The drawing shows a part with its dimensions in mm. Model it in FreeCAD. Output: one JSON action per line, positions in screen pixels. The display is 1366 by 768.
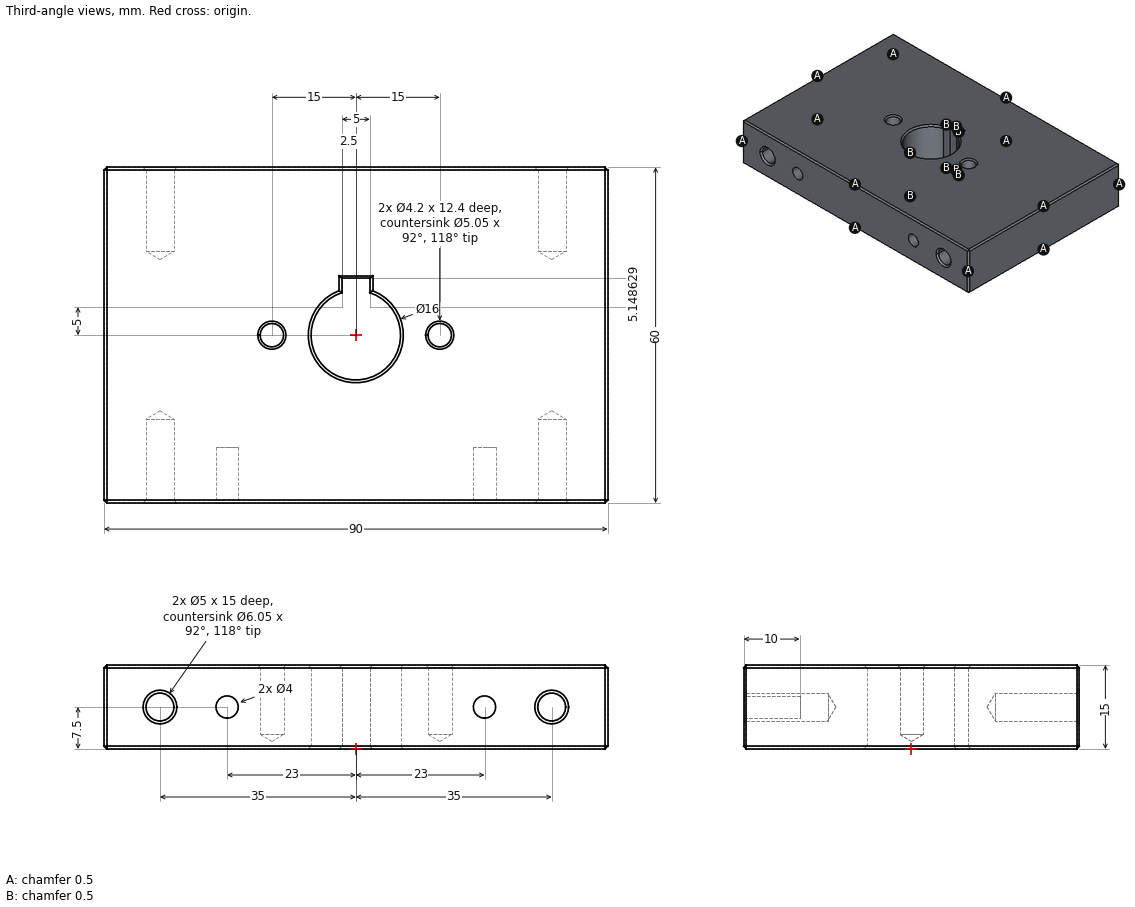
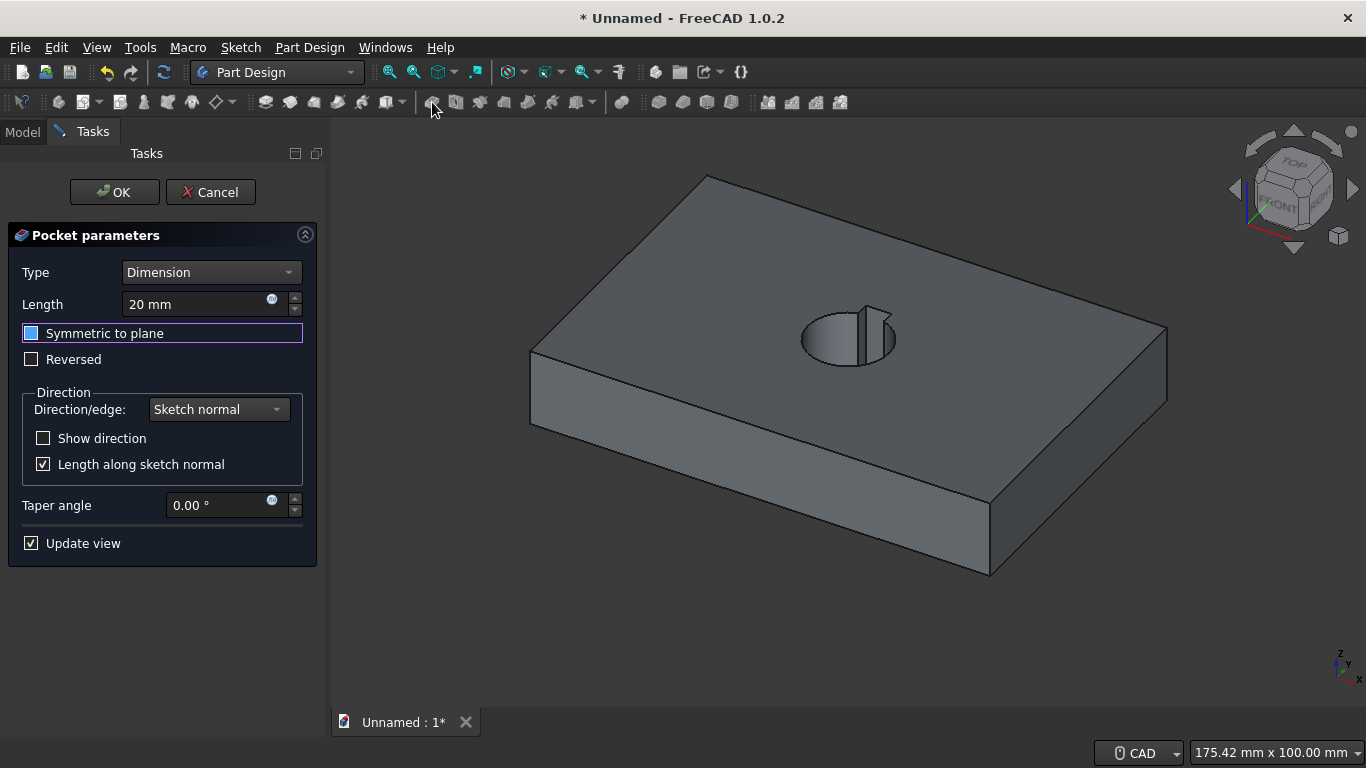
{"action": "left_click", "coordinate": [115, 192]}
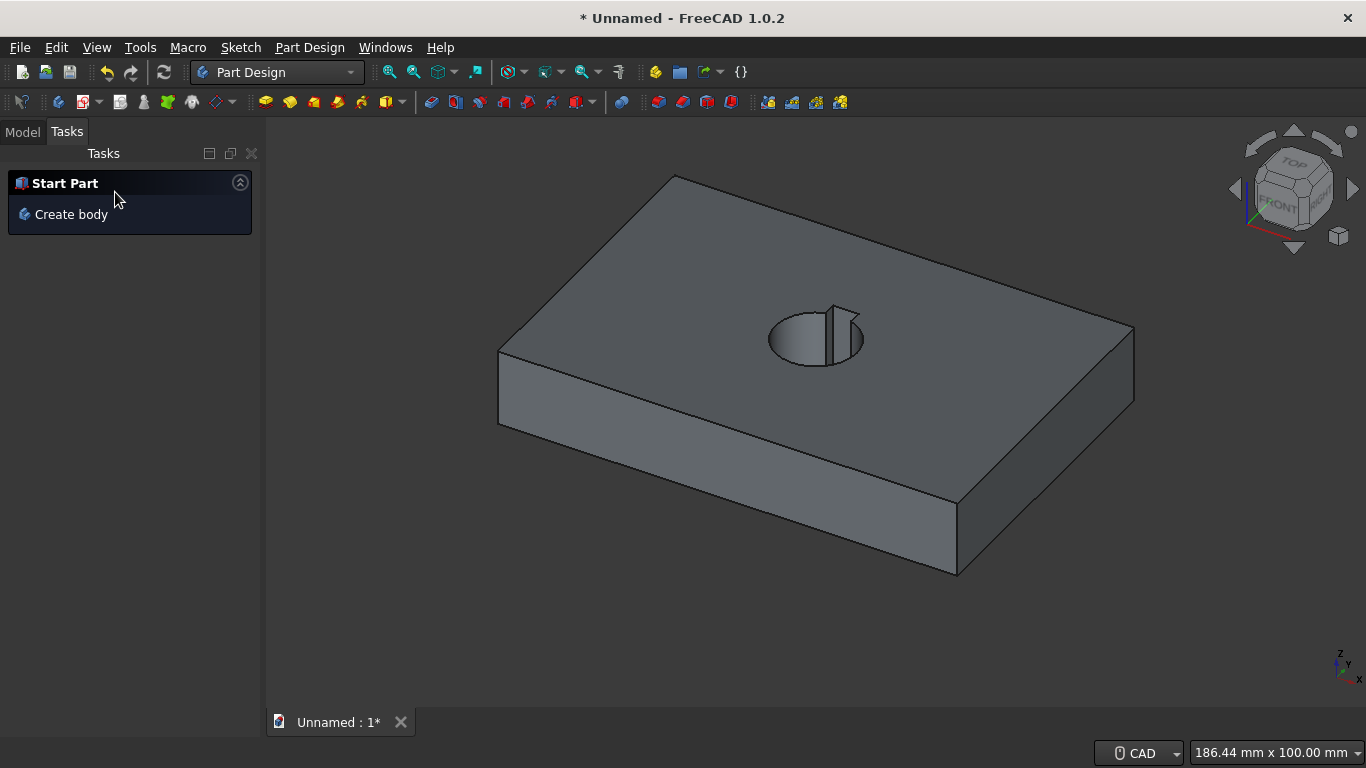
{"action": "left_click", "coordinate": [659, 320]}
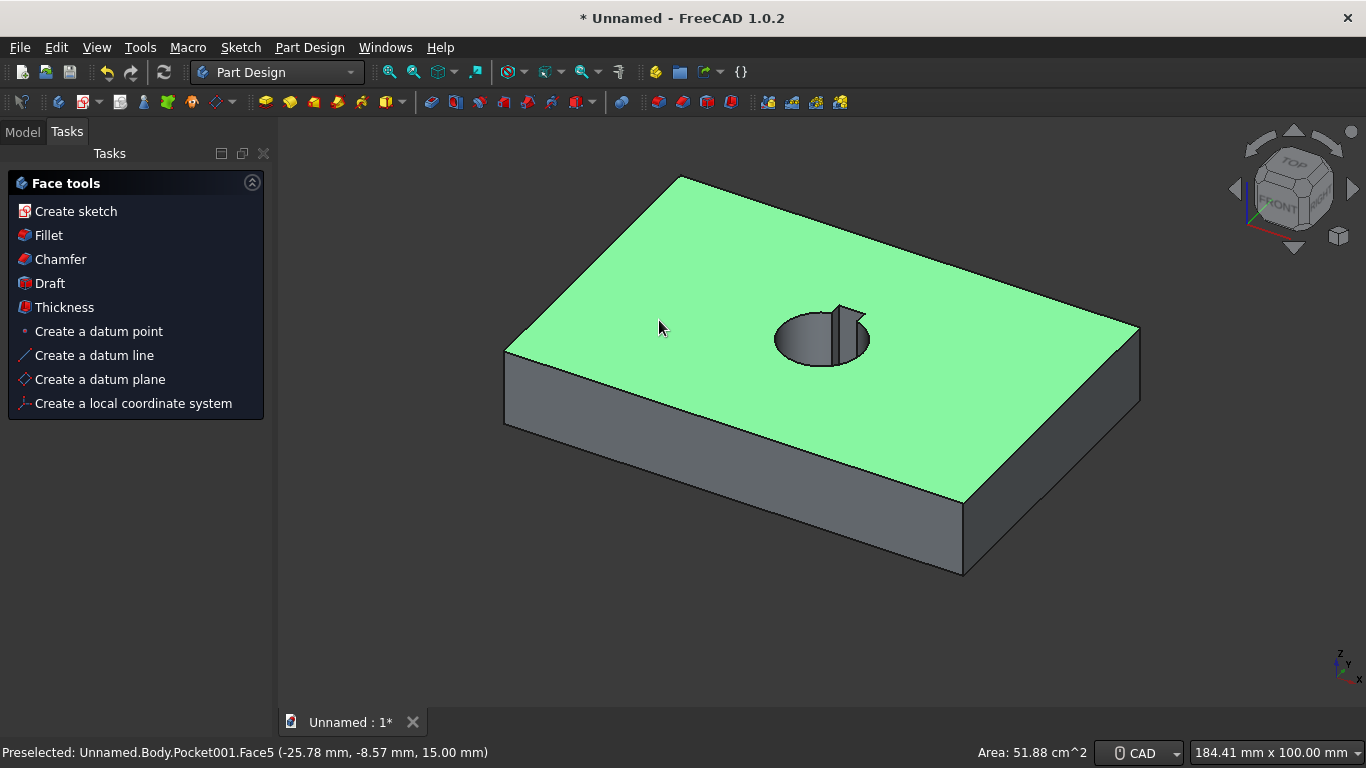
{"action": "left_click", "coordinate": [84, 102]}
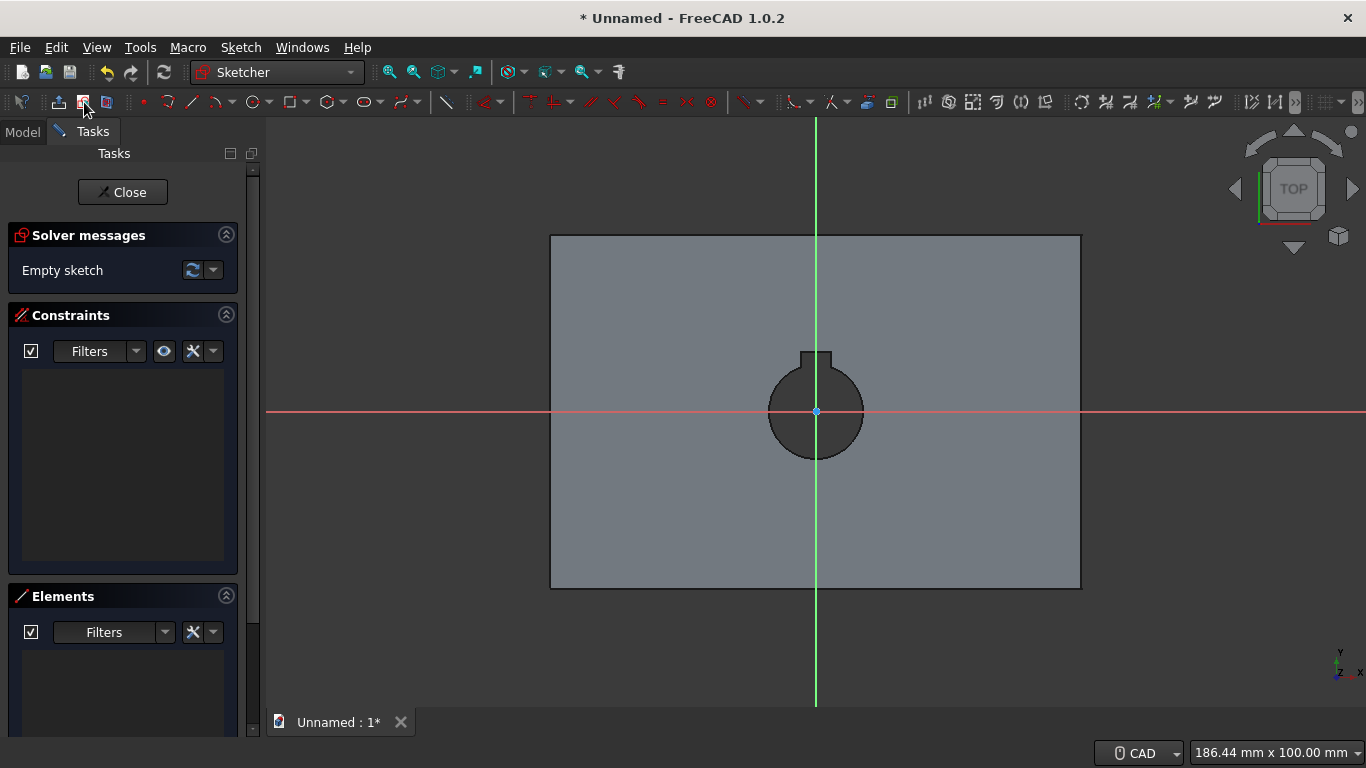
{"action": "scroll", "coordinate": [846, 412], "scroll_direction": "up", "scroll_amount": 6}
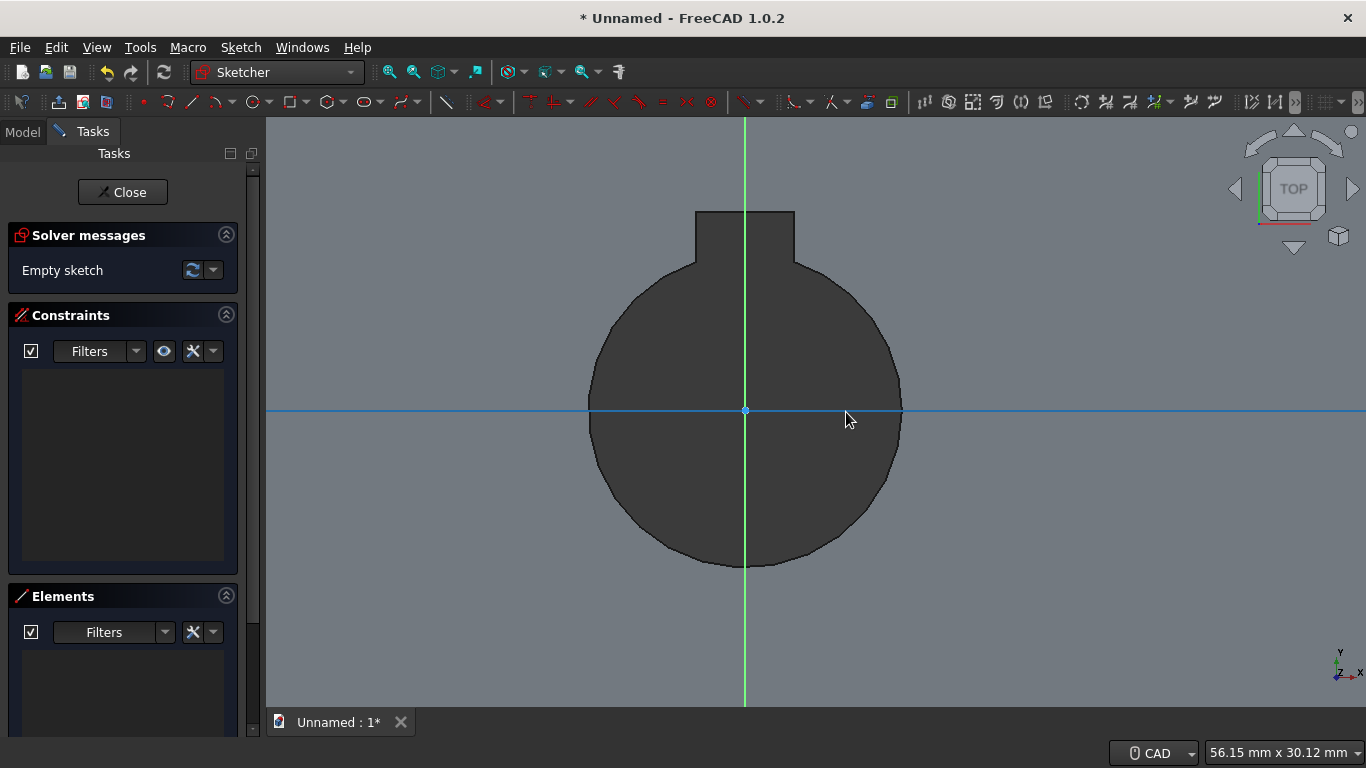
{"action": "left_click", "coordinate": [254, 102]}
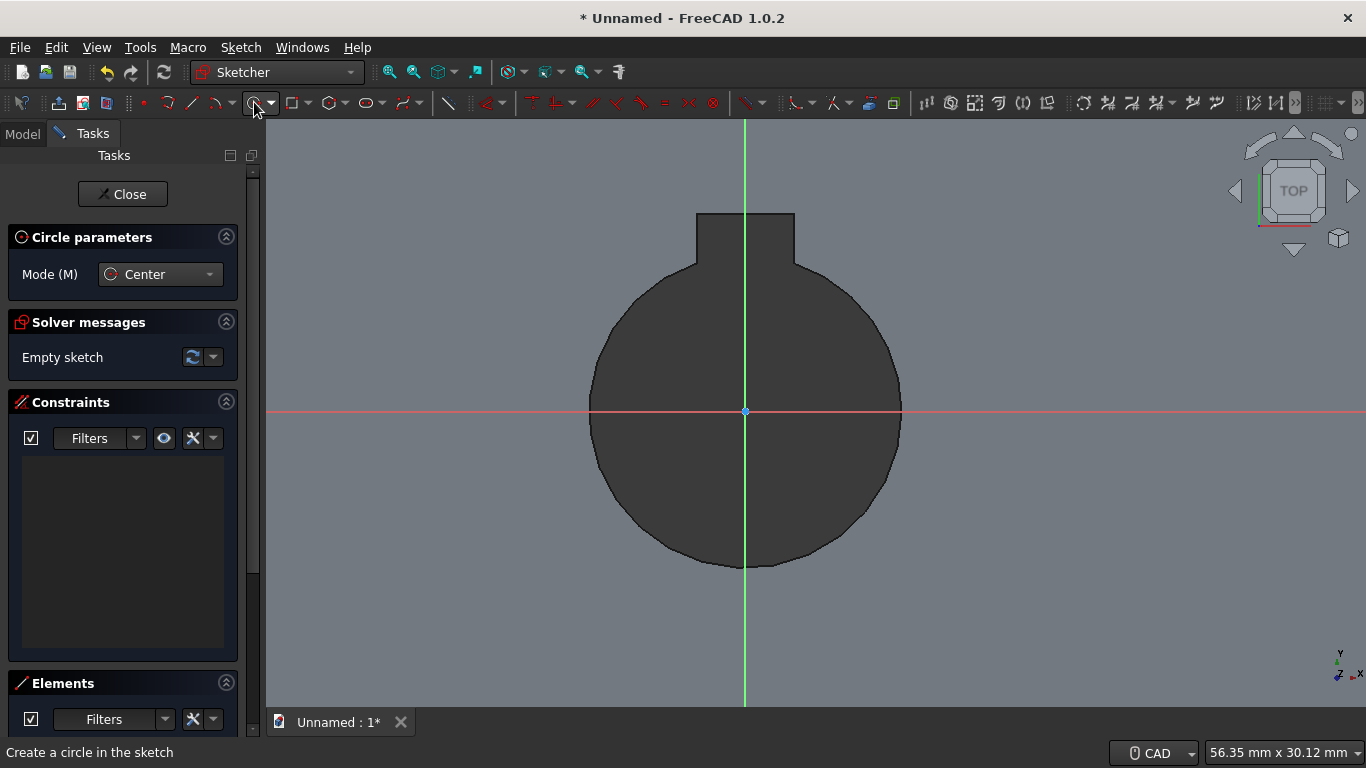
{"action": "left_click", "coordinate": [1038, 412]}
{"action": "mouse_move", "coordinate": [1067, 383]}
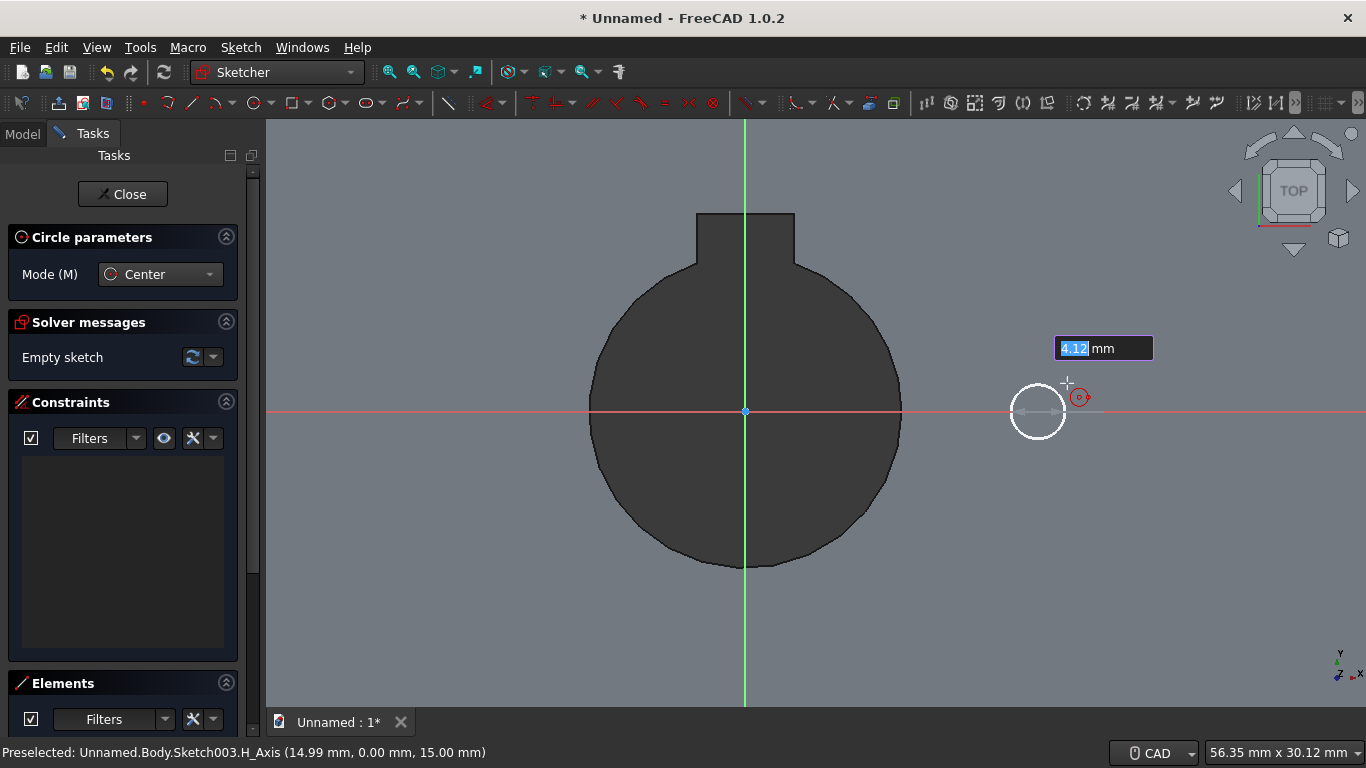
{"action": "type", "text": "4.2"}
{"action": "key", "text": "Return"}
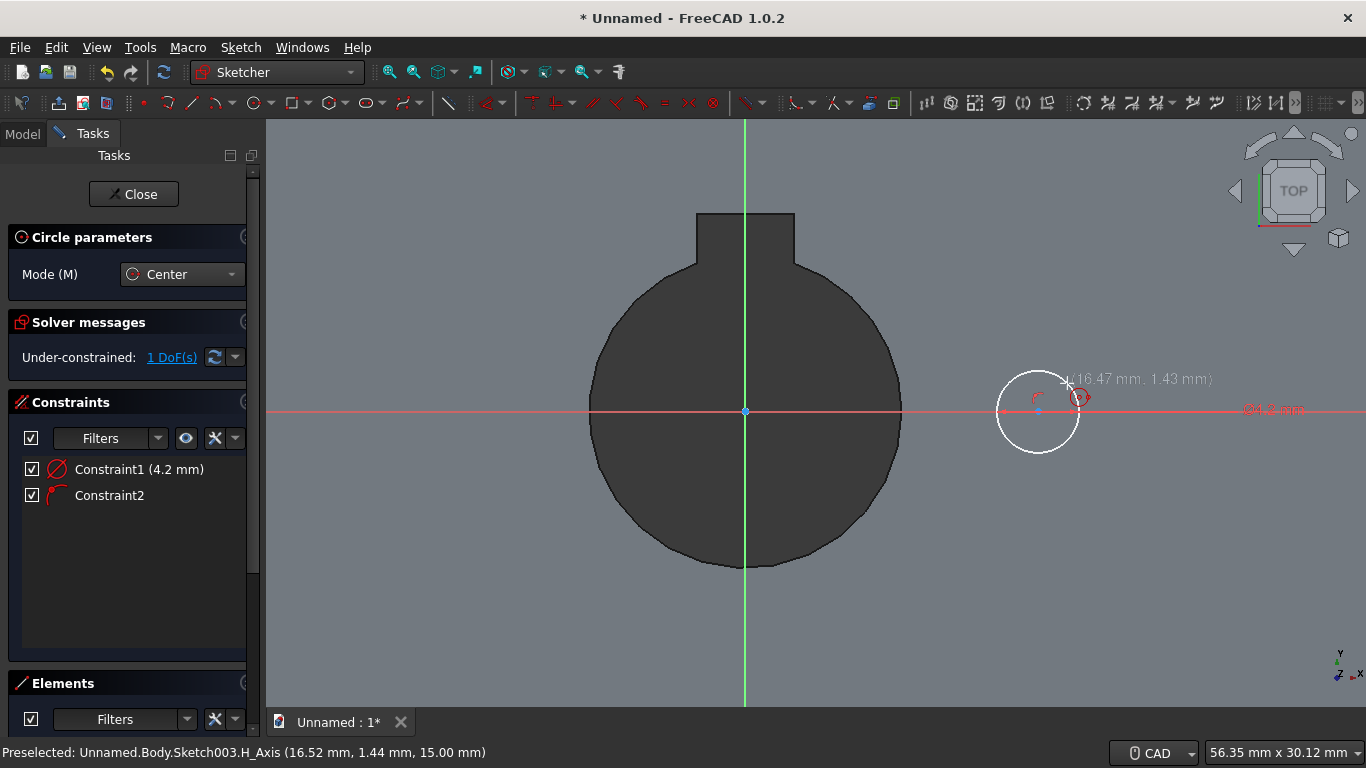
{"action": "left_click", "coordinate": [453, 412]}
{"action": "mouse_move", "coordinate": [482, 383]}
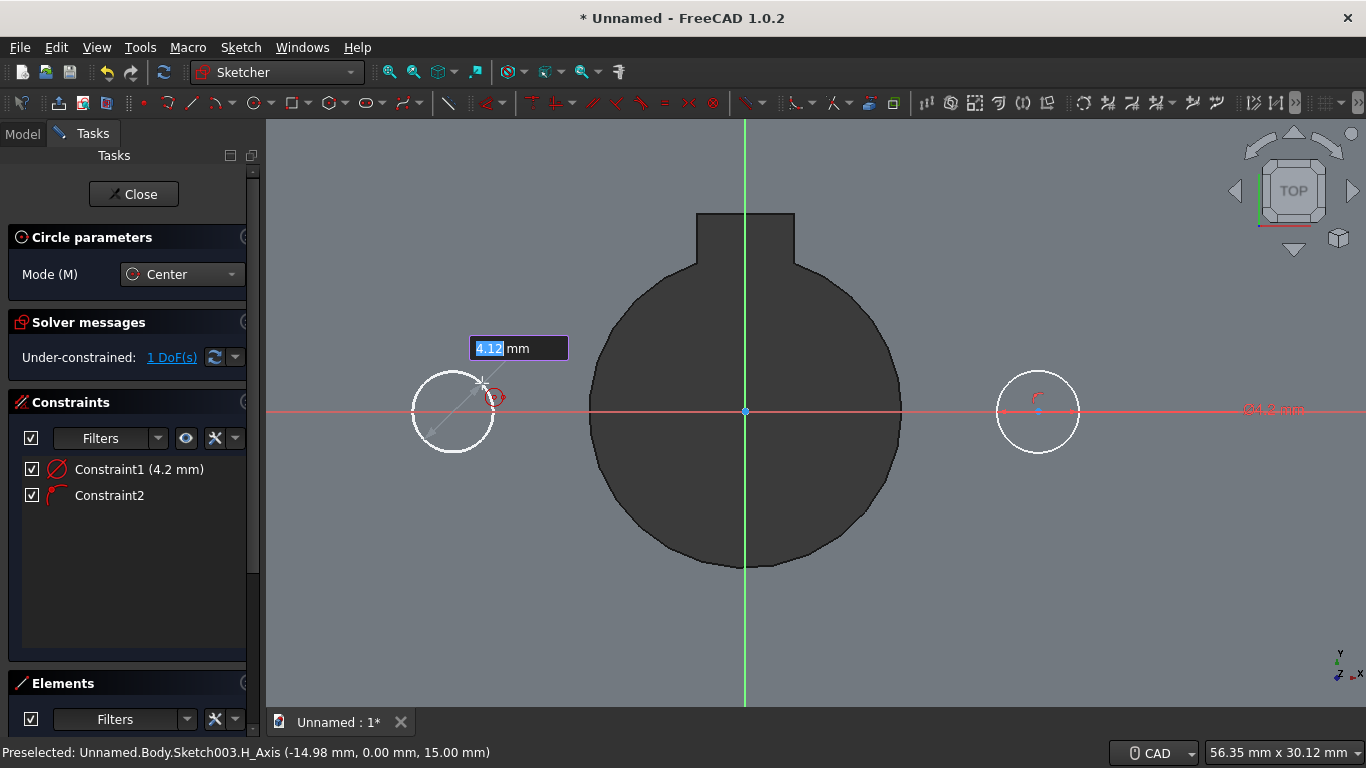
{"action": "type", "text": "4.2"}
{"action": "key", "text": "Return"}
{"action": "key", "text": "Escape"}